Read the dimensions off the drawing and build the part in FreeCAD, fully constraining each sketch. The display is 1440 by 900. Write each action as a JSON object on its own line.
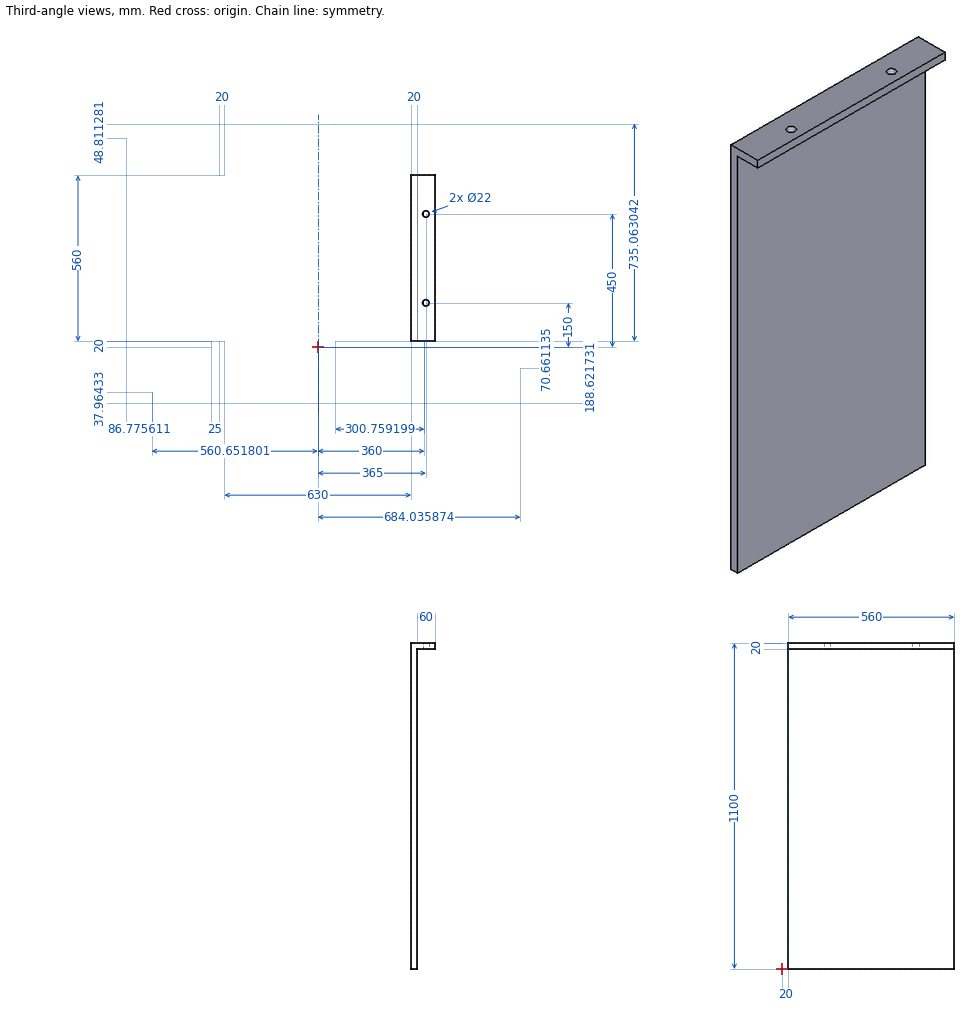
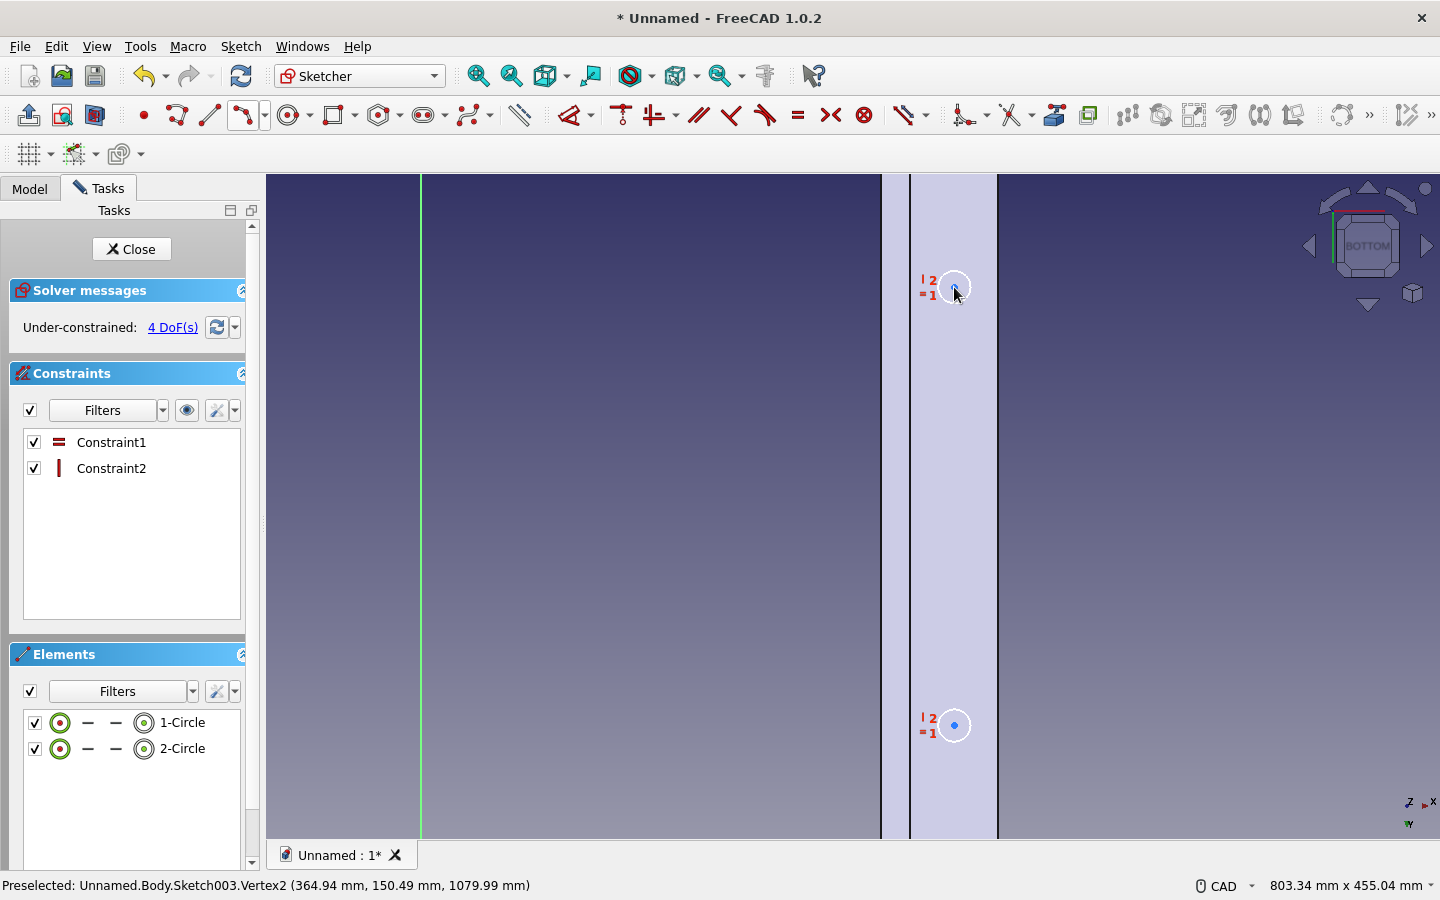
{"action": "left_click", "coordinate": [568, 116]}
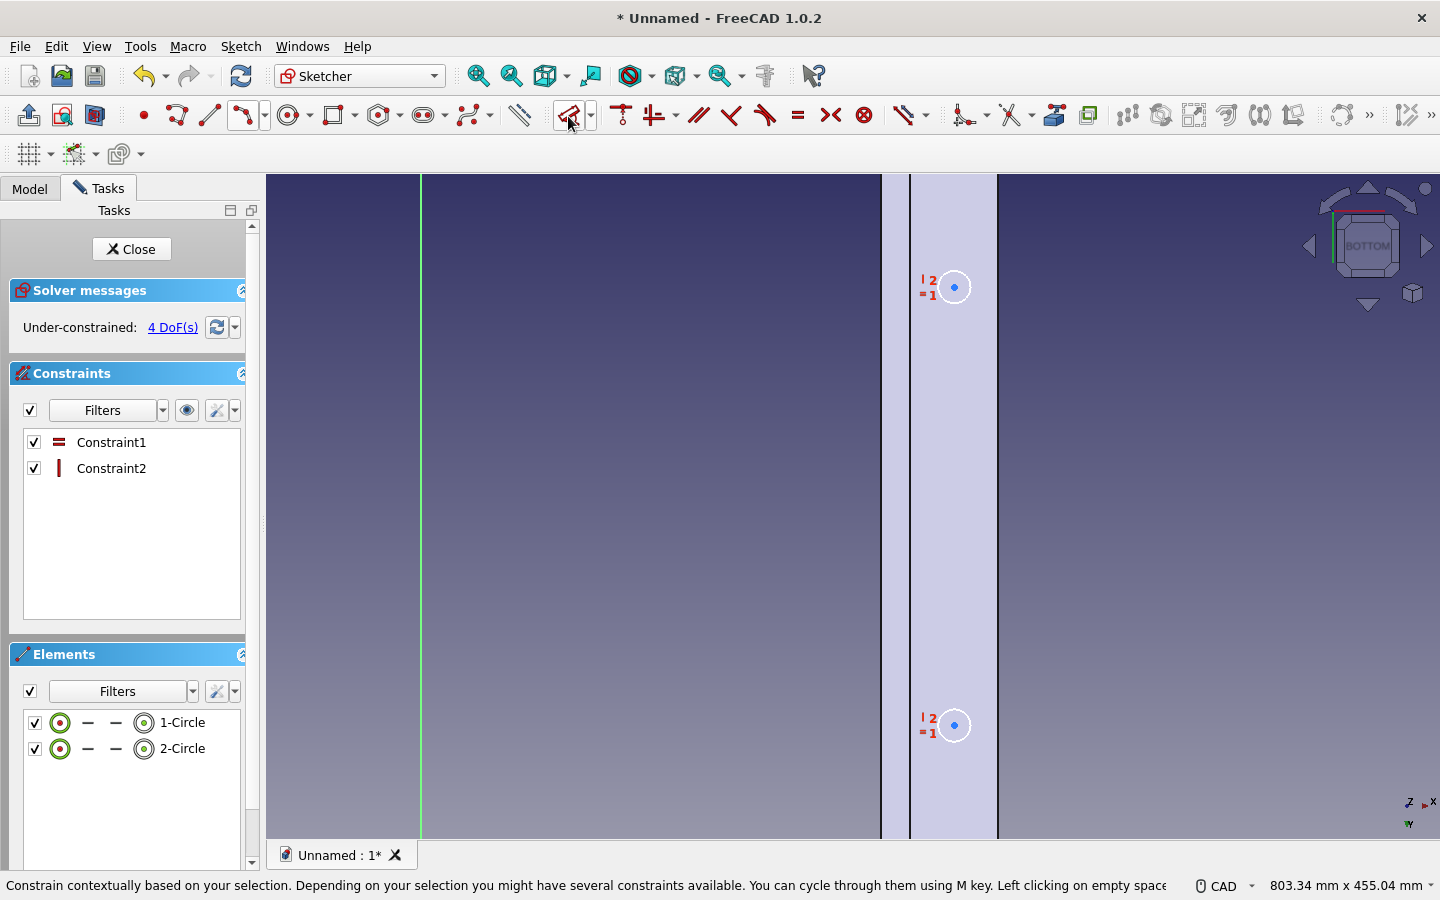
{"action": "scroll", "coordinate": [966, 714], "scroll_direction": "up", "scroll_amount": 2}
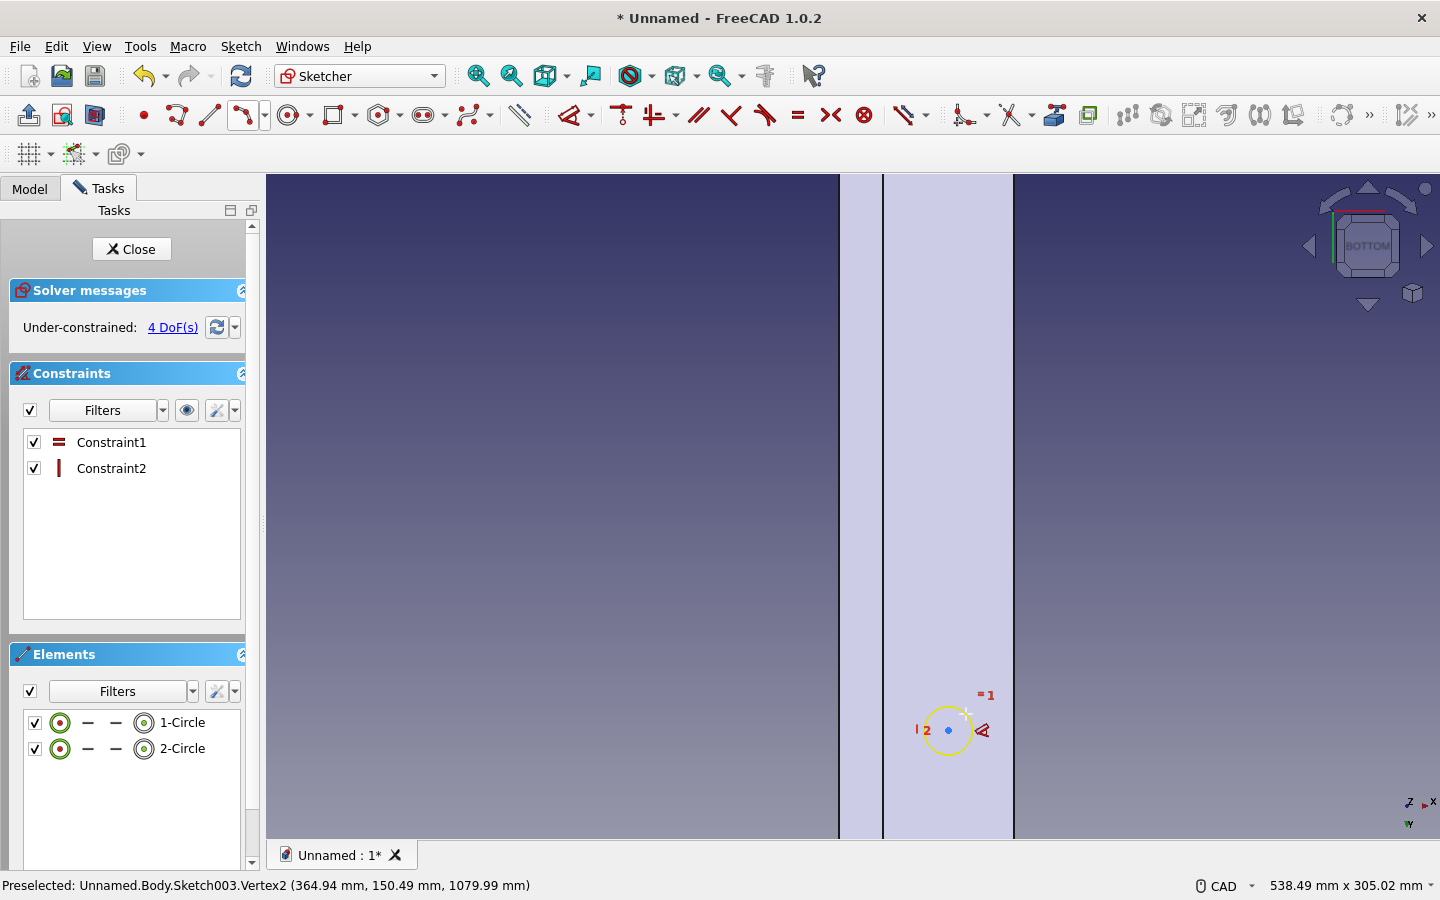
{"action": "left_click", "coordinate": [965, 714]}
{"action": "left_click", "coordinate": [987, 691]}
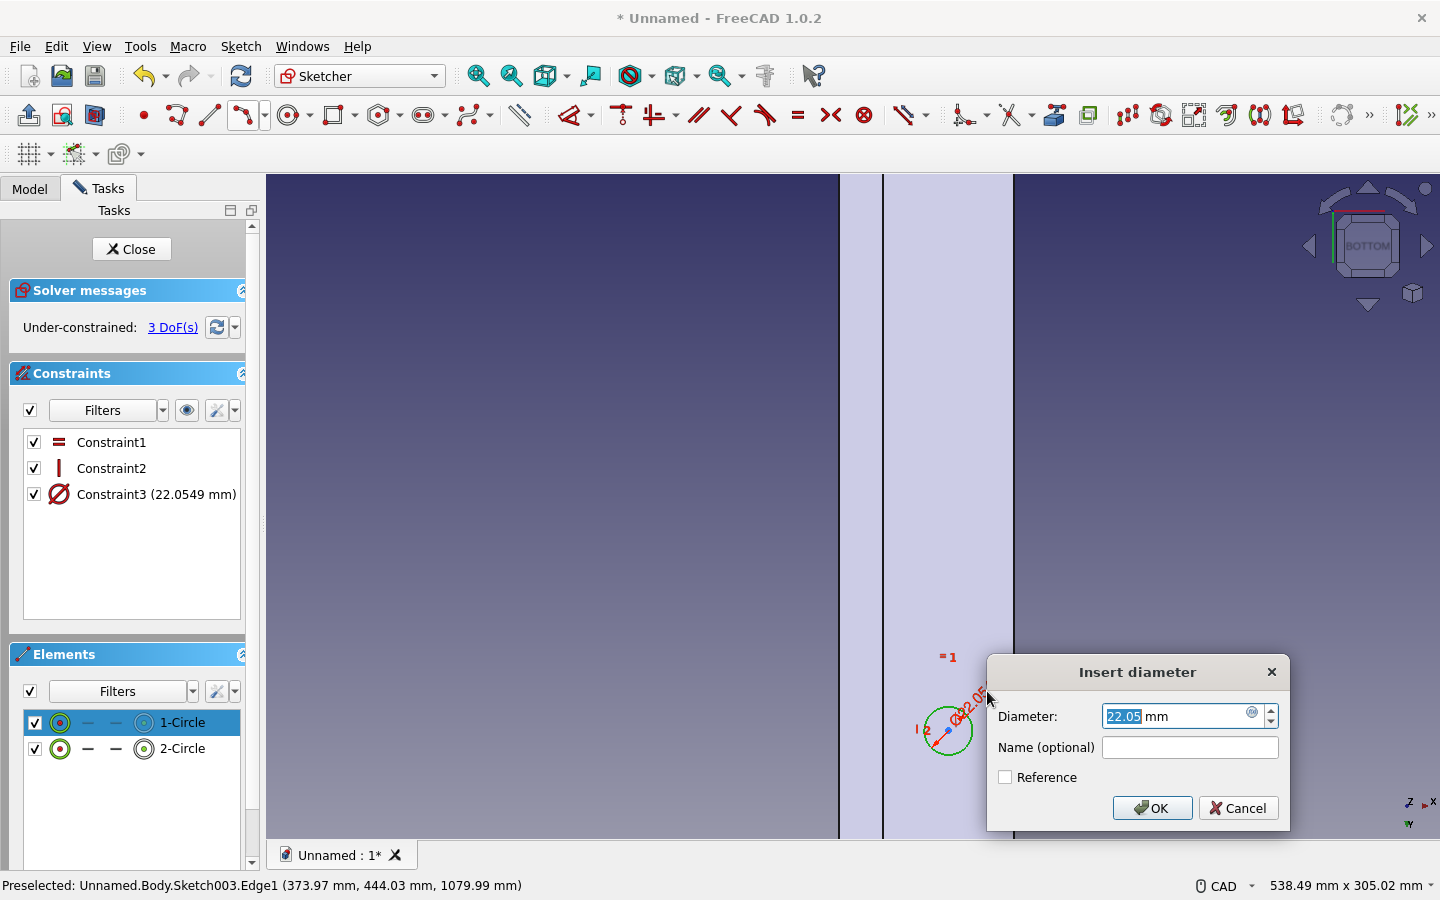
{"action": "type", "text": "22"}
{"action": "key", "text": "Return"}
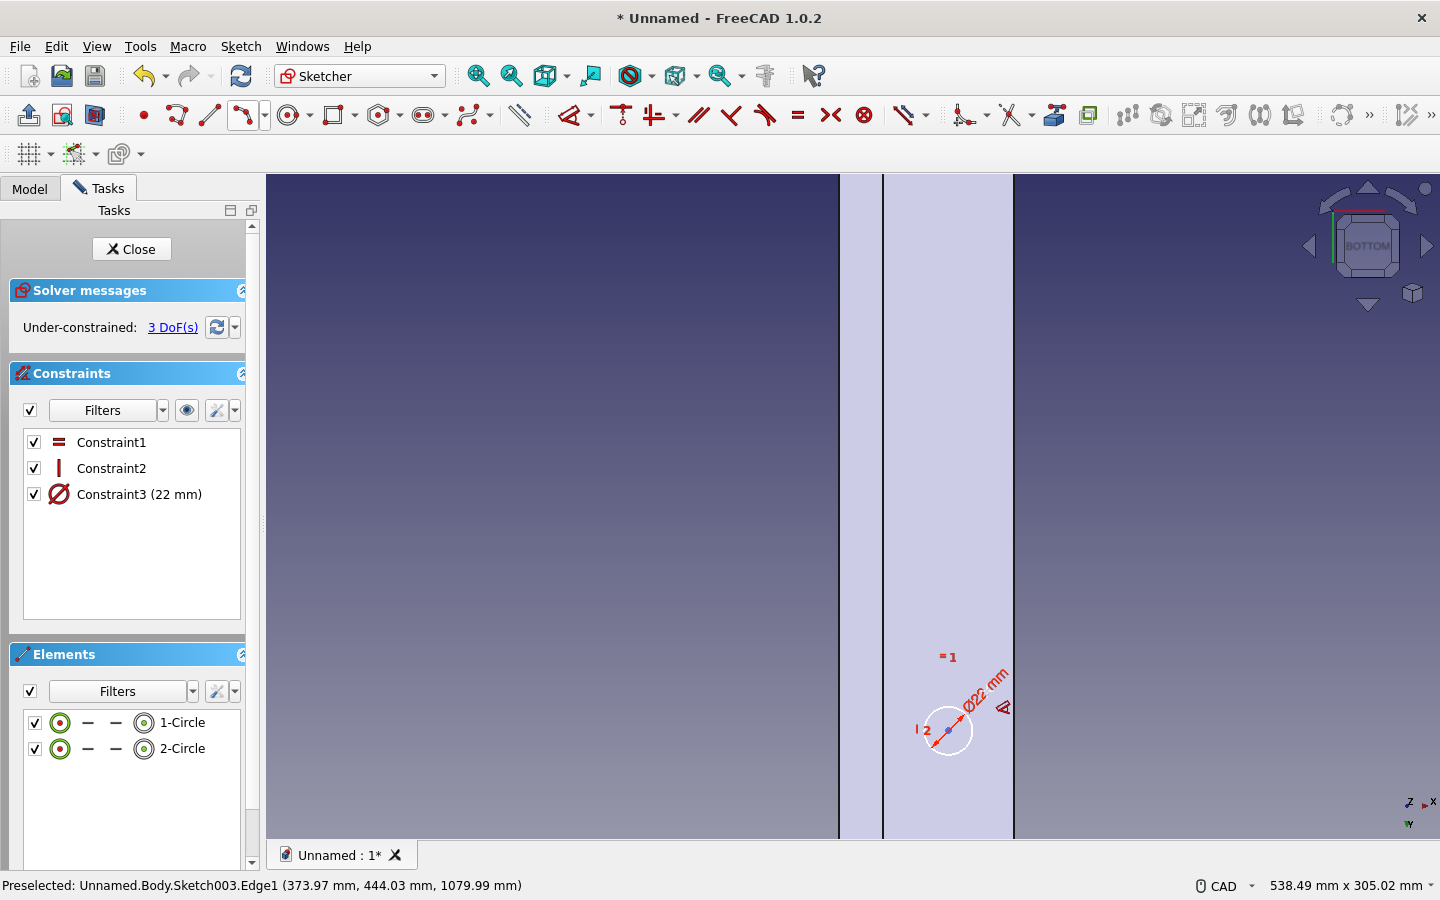
{"action": "left_click", "coordinate": [948, 731]}
{"action": "left_click", "coordinate": [621, 765]}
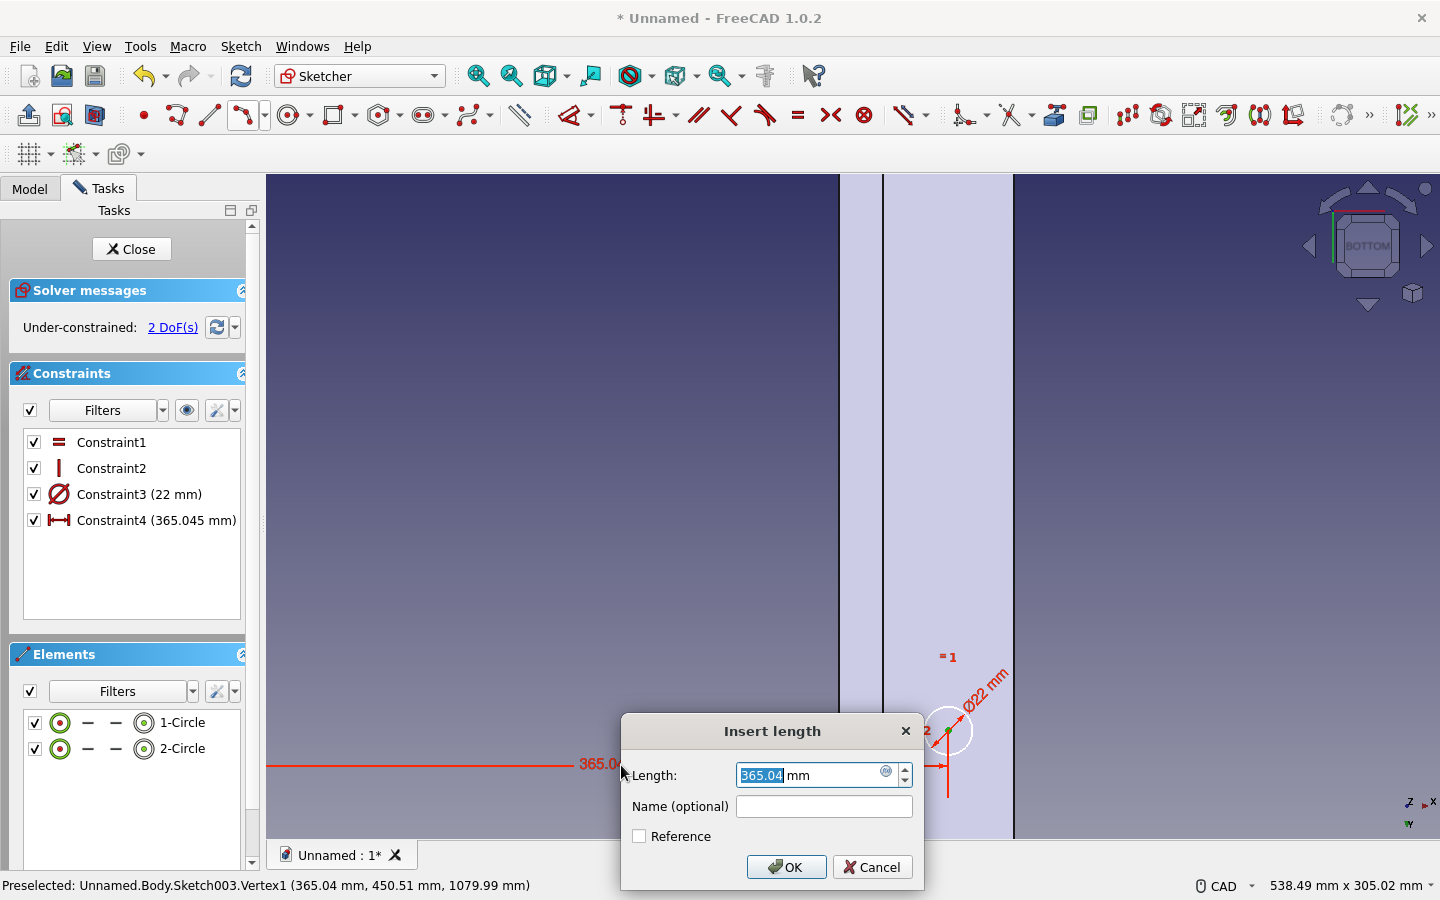
{"action": "type", "text": "365"}
{"action": "key", "text": "Return"}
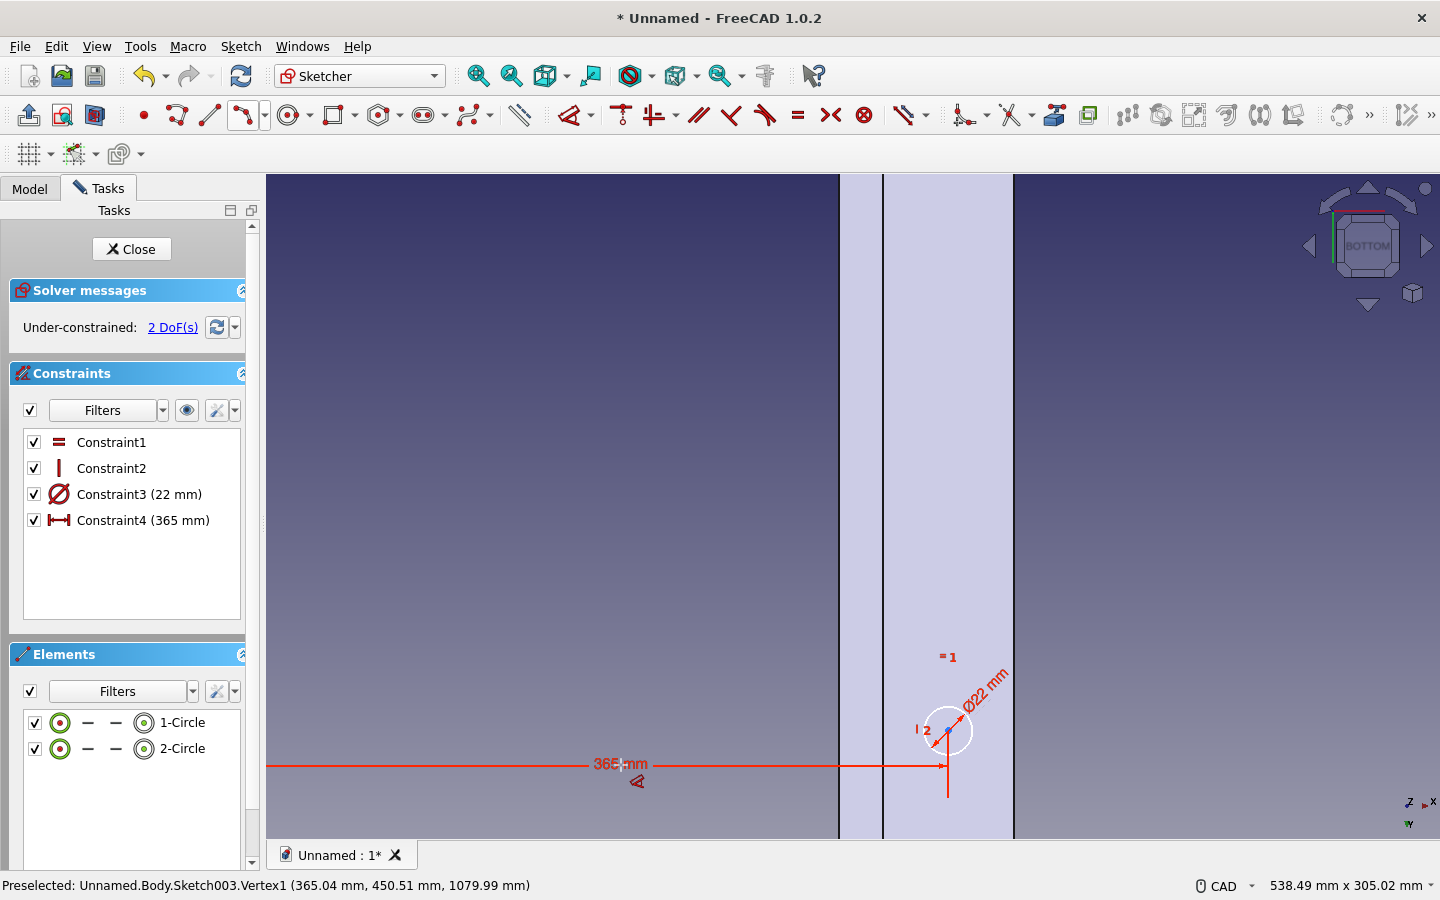
{"action": "left_click", "coordinate": [948, 731]}
{"action": "left_click", "coordinate": [982, 466]}